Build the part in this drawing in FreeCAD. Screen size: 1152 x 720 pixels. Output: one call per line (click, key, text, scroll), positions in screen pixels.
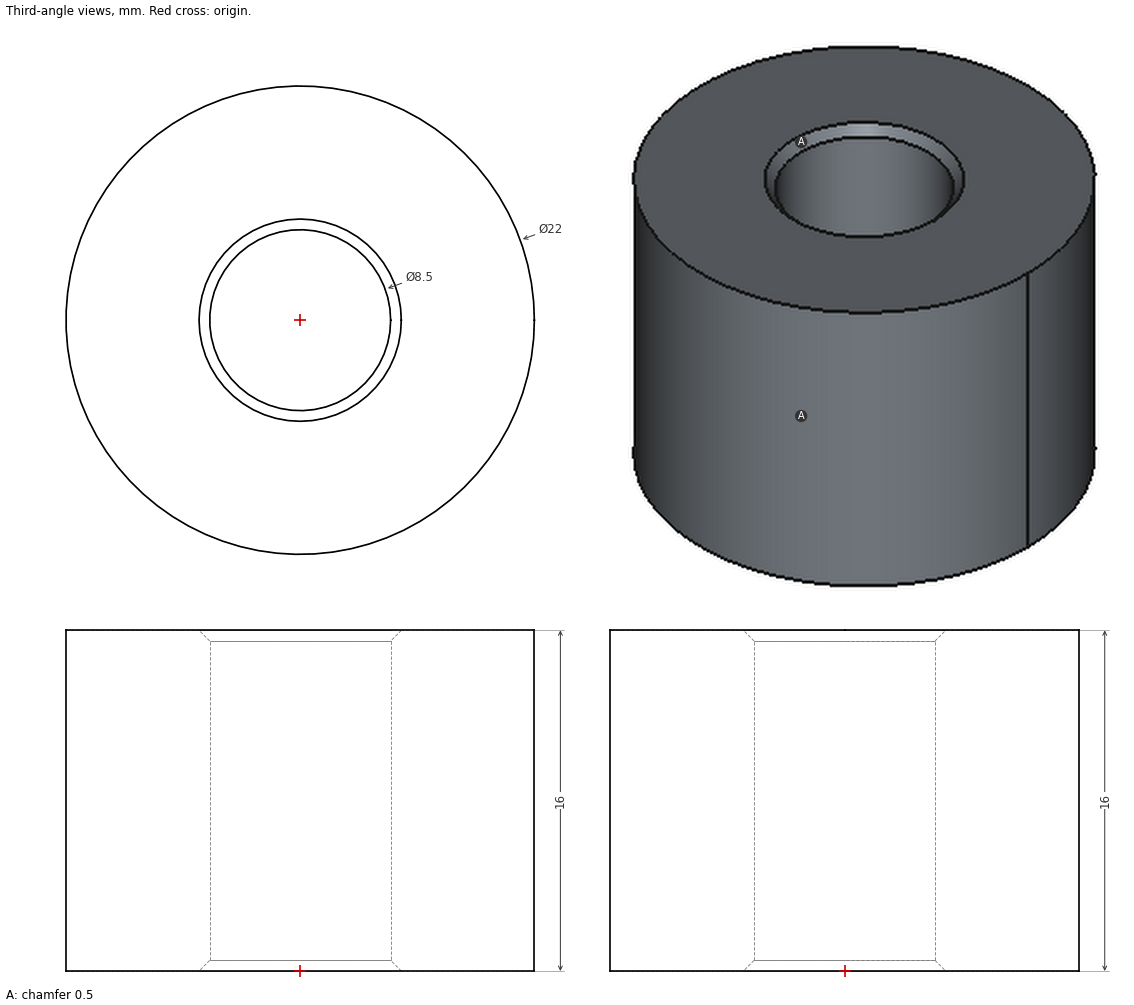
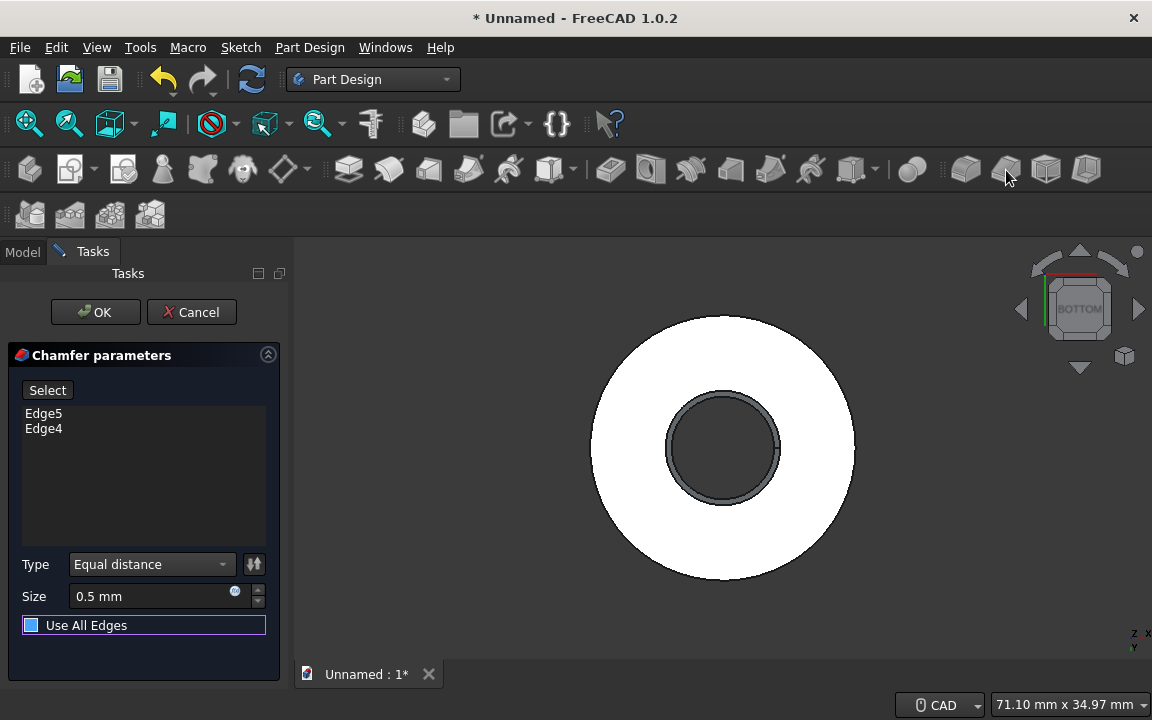
click(96, 312)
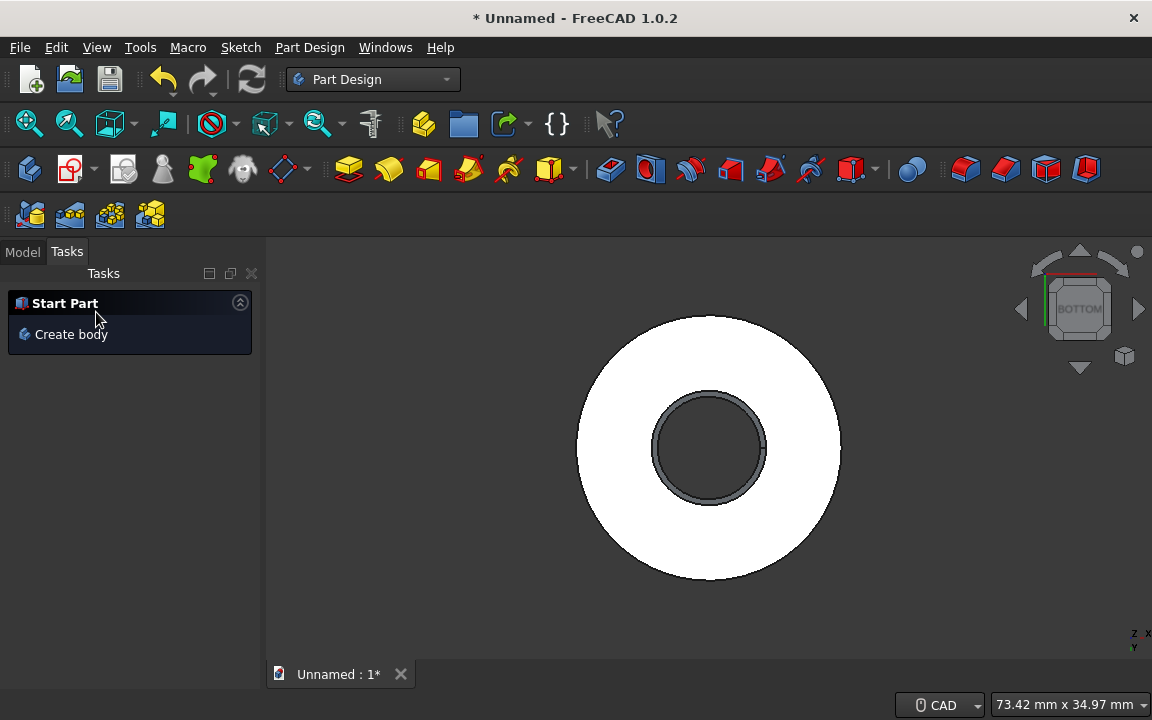
key(0)